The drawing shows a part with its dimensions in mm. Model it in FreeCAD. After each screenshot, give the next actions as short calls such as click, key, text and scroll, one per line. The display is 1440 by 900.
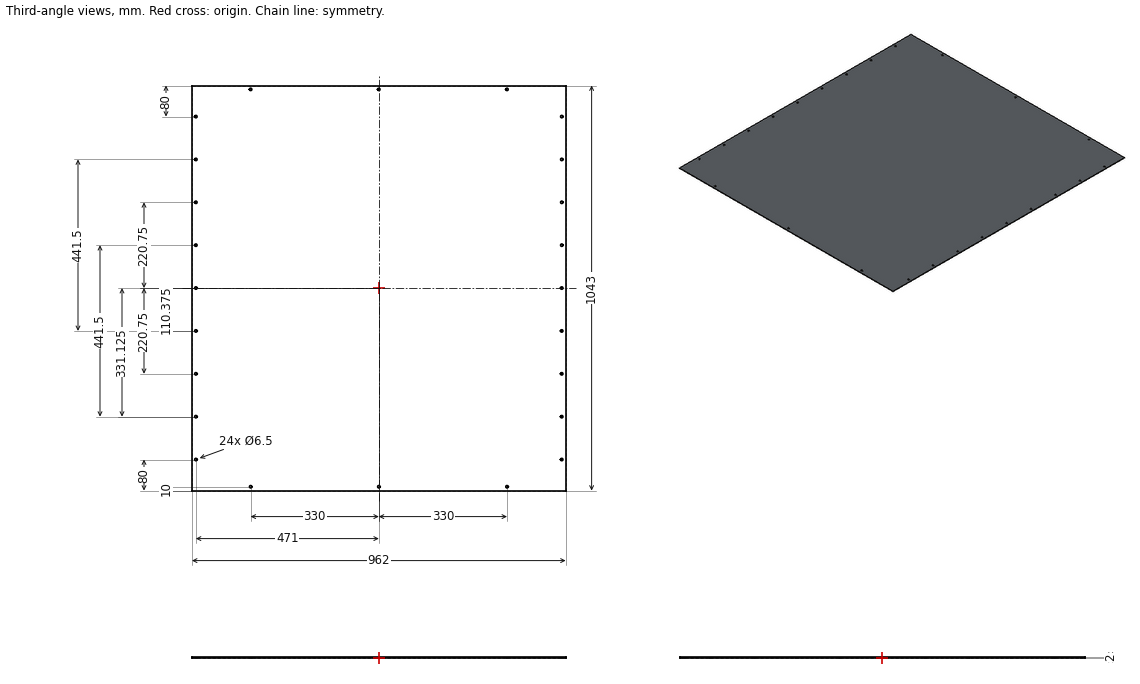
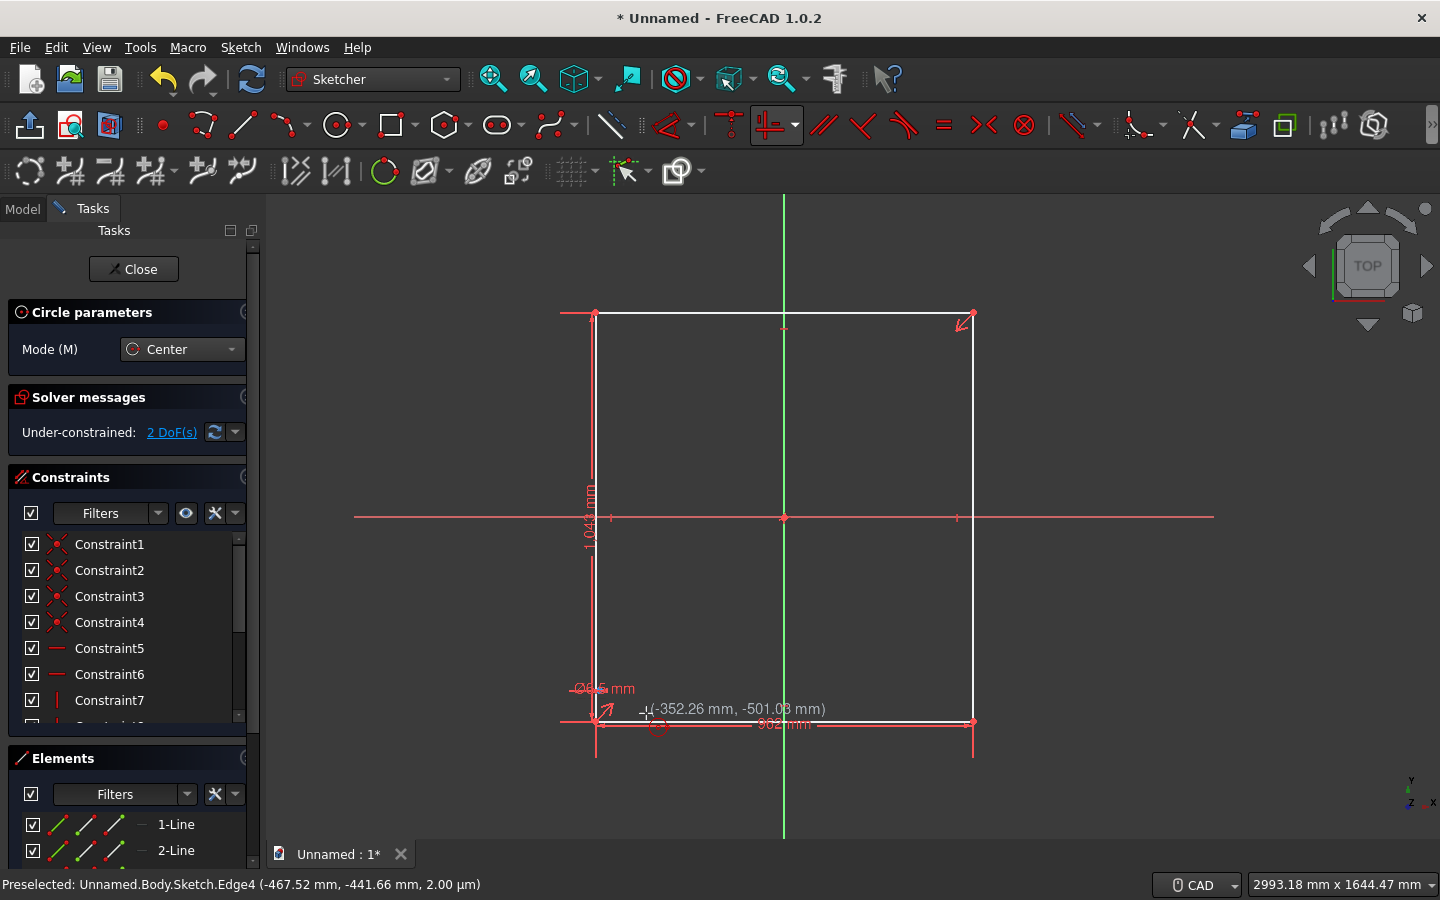
scroll(655, 718, up, 7)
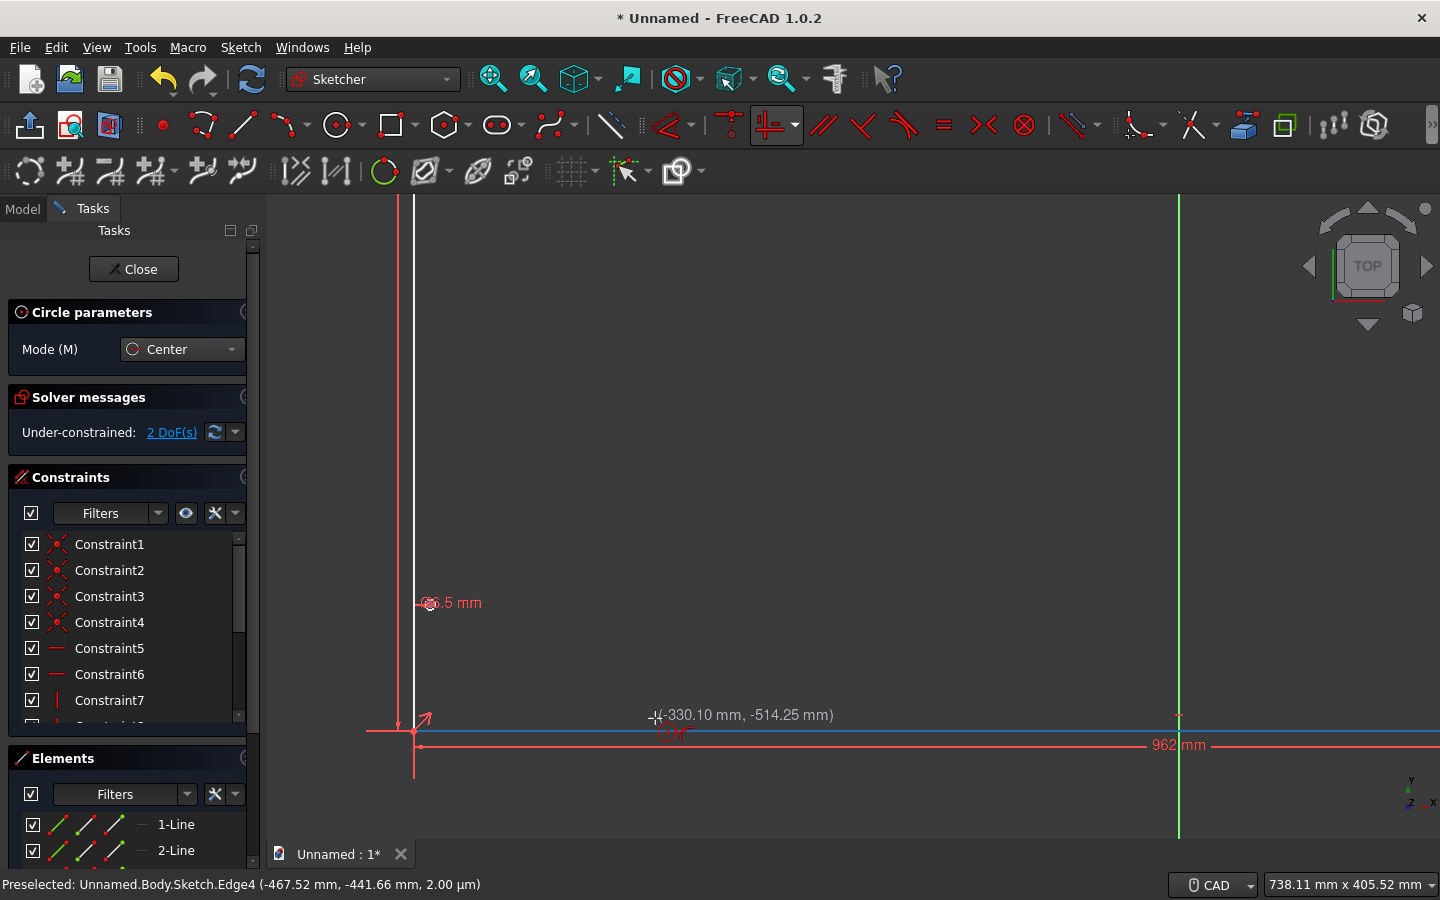
click(654, 715)
move(658, 712)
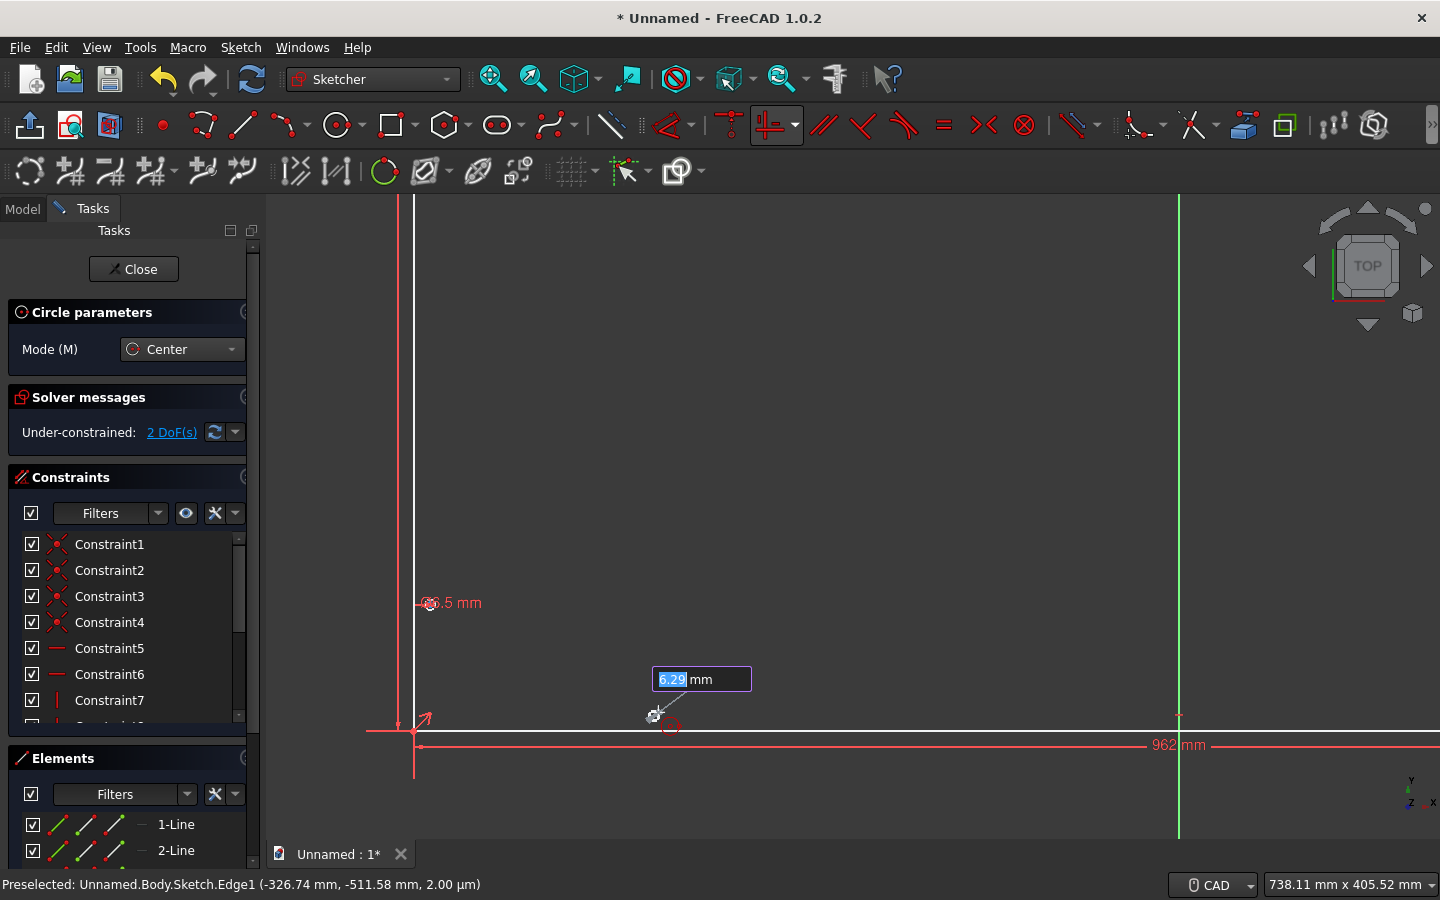
text(6.5)
key(Return)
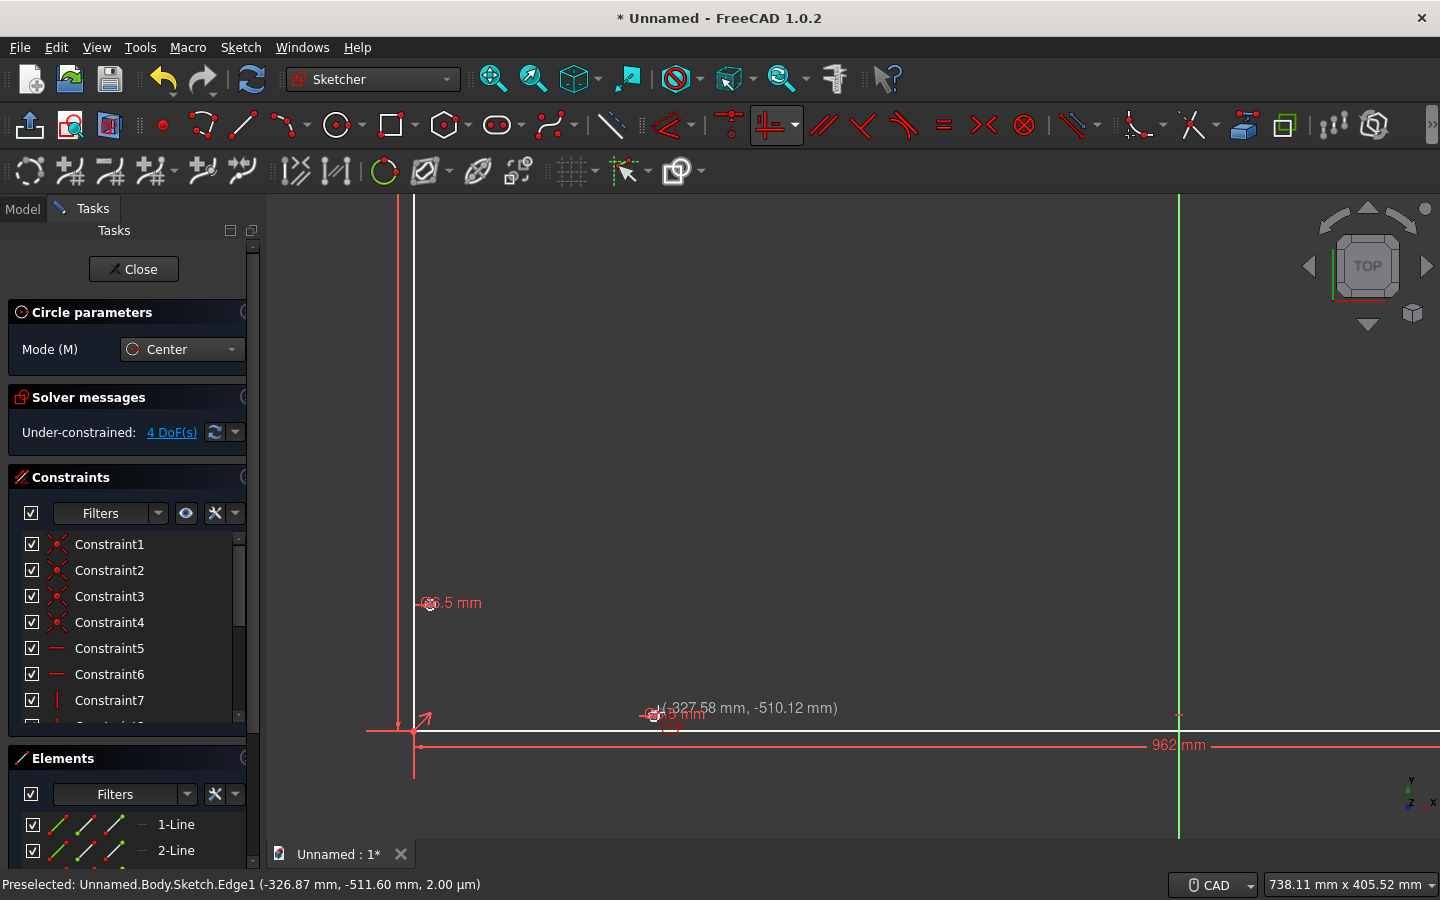
scroll(430, 428, up, 8)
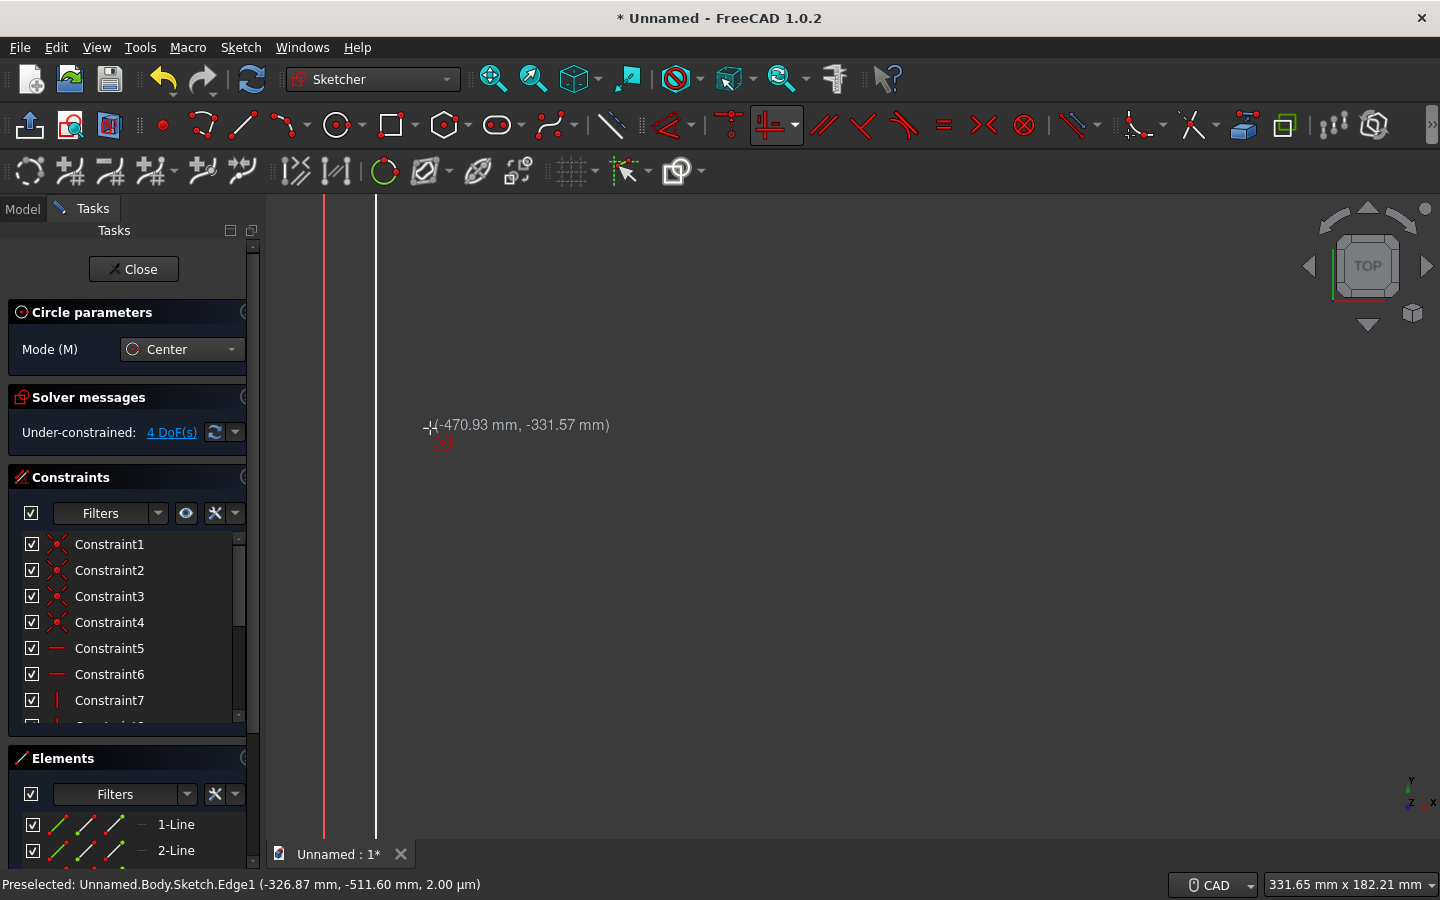
scroll(609, 658, down, 15)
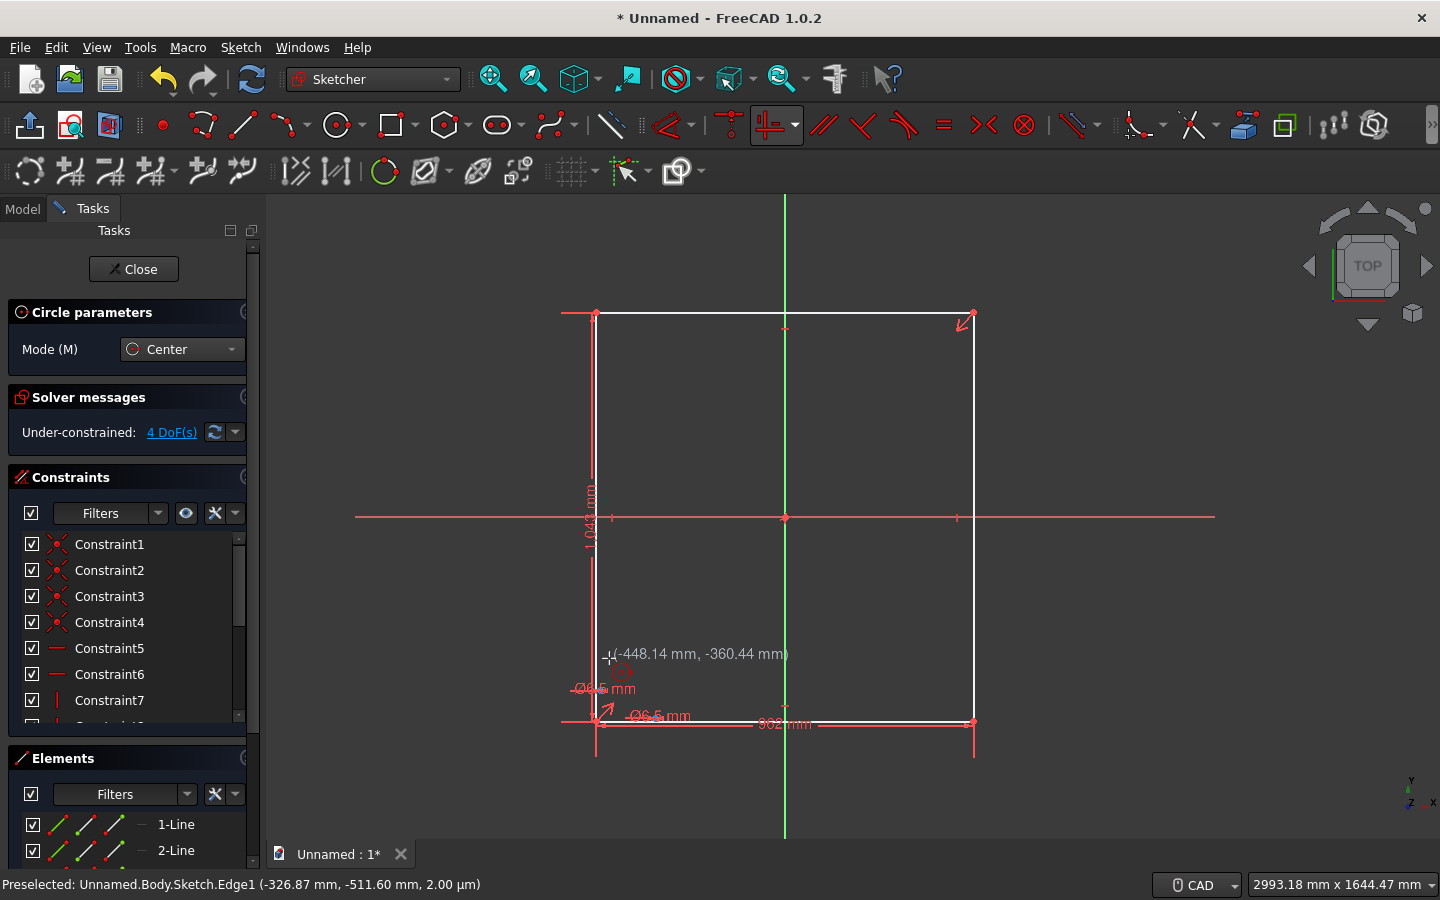
scroll(600, 647, up, 7)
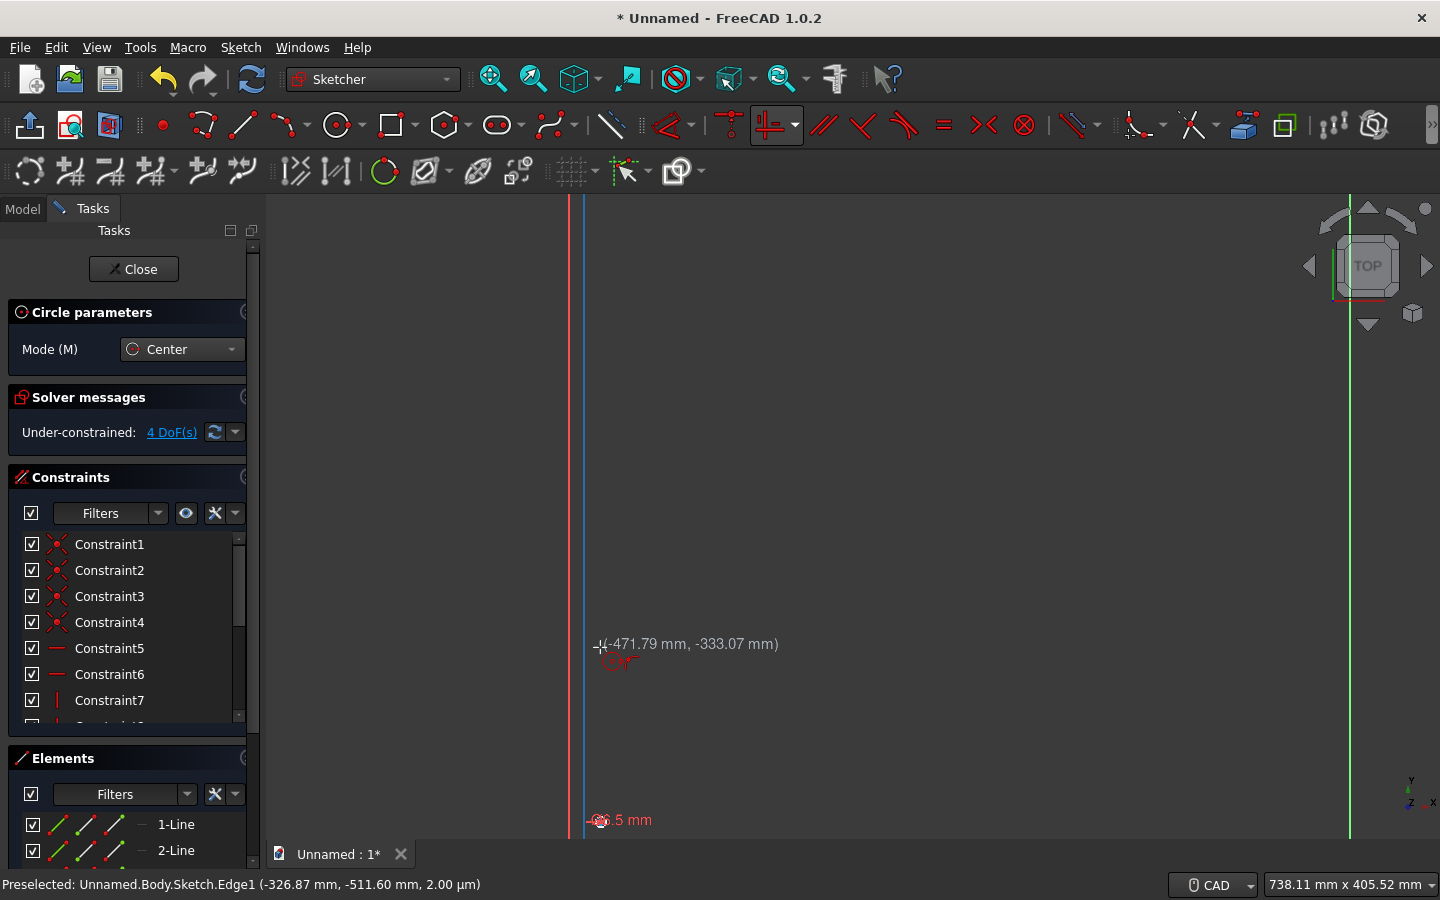
click(600, 646)
move(604, 642)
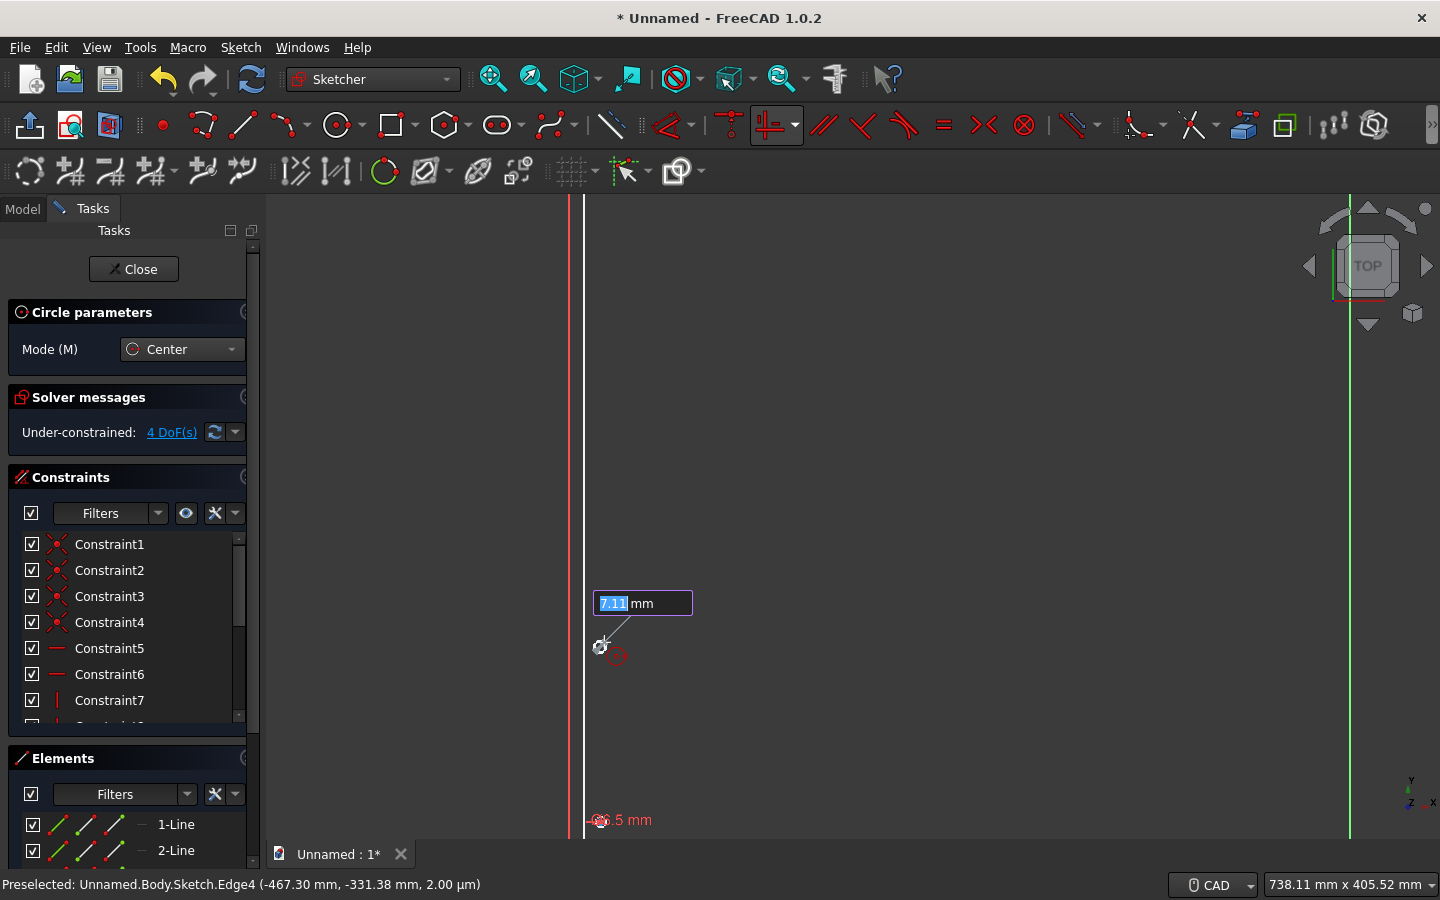
text(6.5)
key(Return)